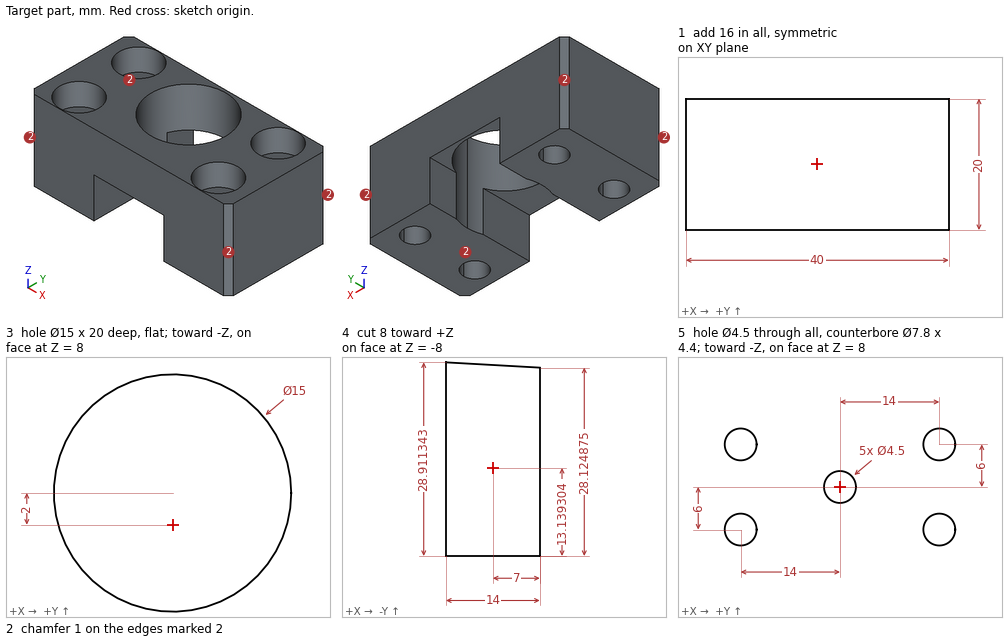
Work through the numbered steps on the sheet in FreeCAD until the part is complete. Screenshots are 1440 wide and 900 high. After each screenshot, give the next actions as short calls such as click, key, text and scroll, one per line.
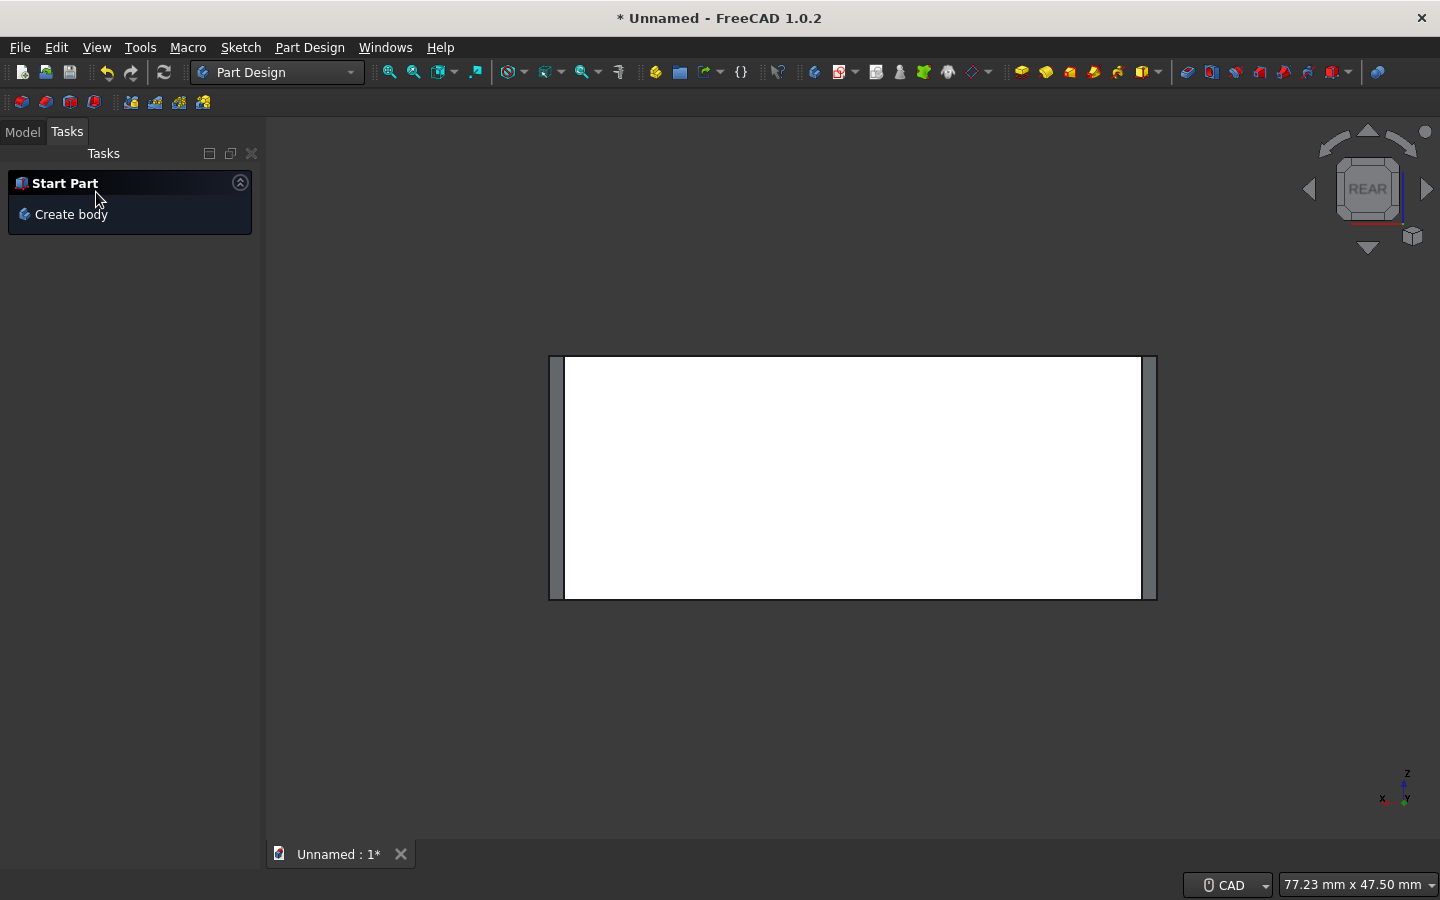
key(0)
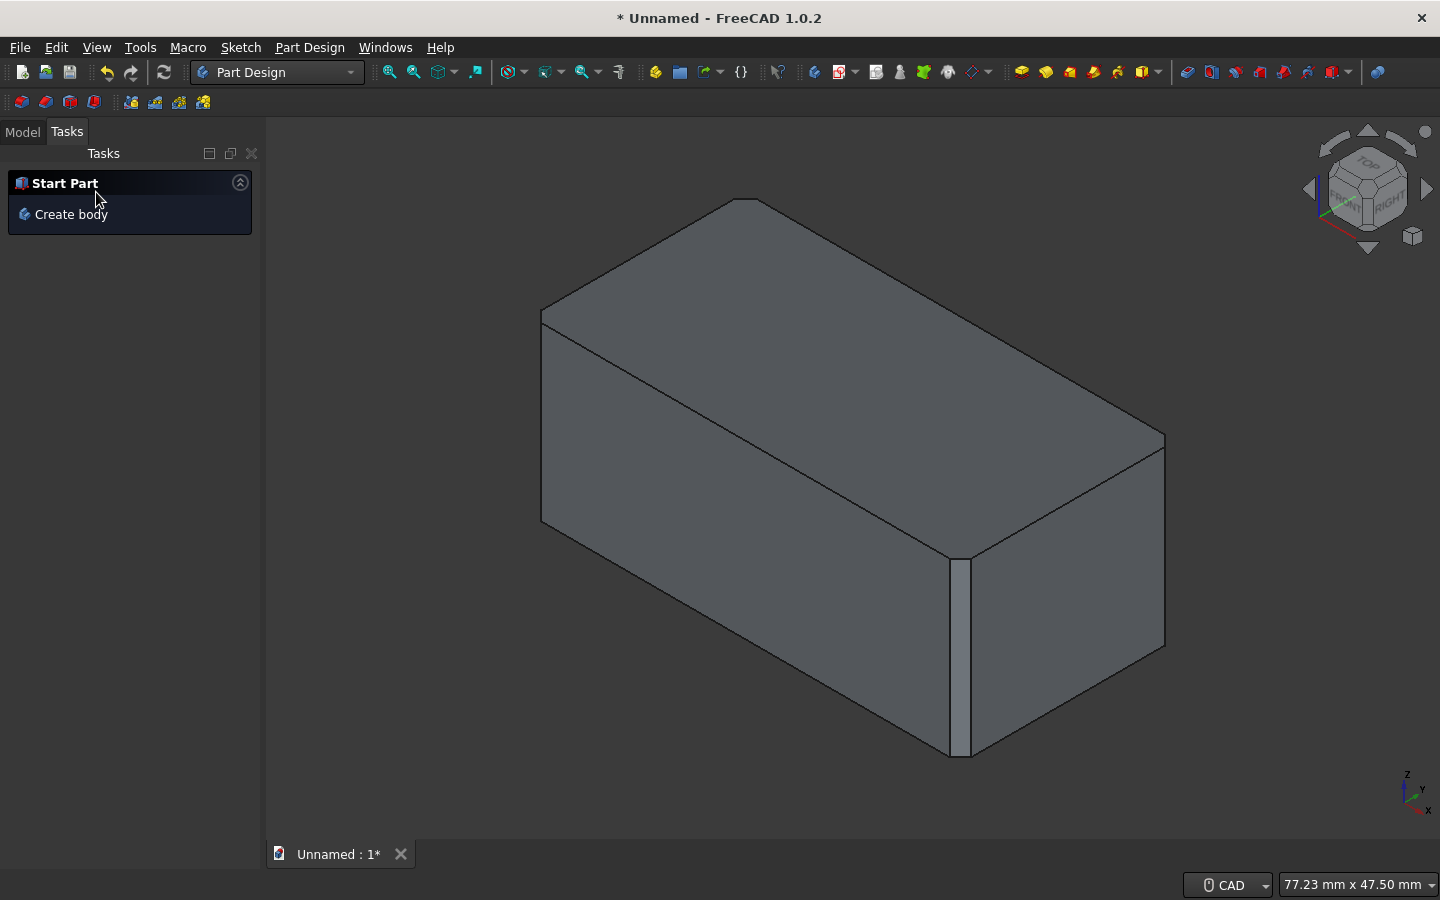
click(914, 413)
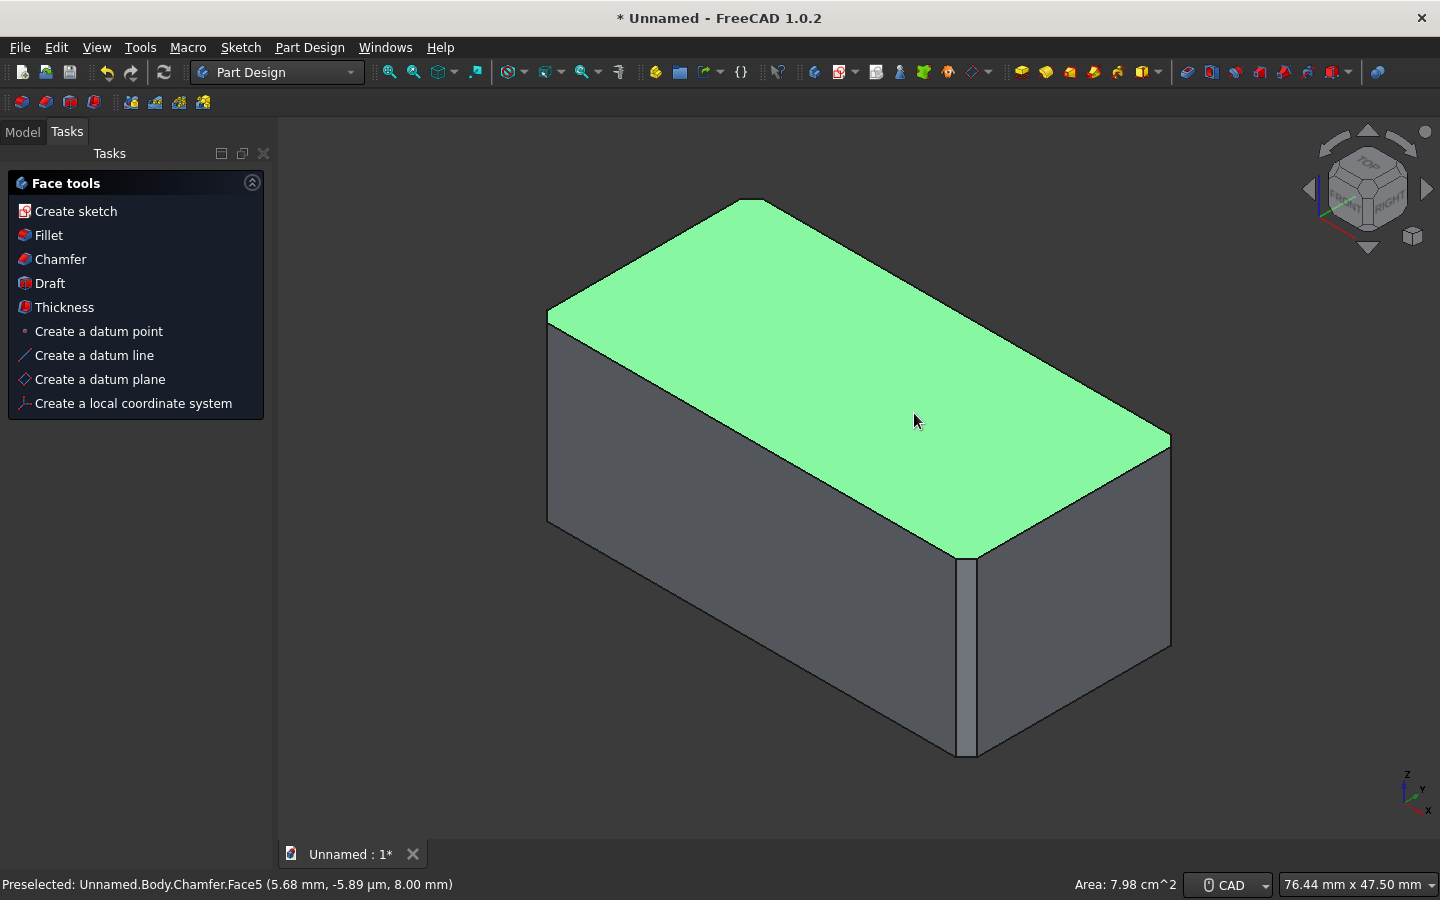
click(840, 72)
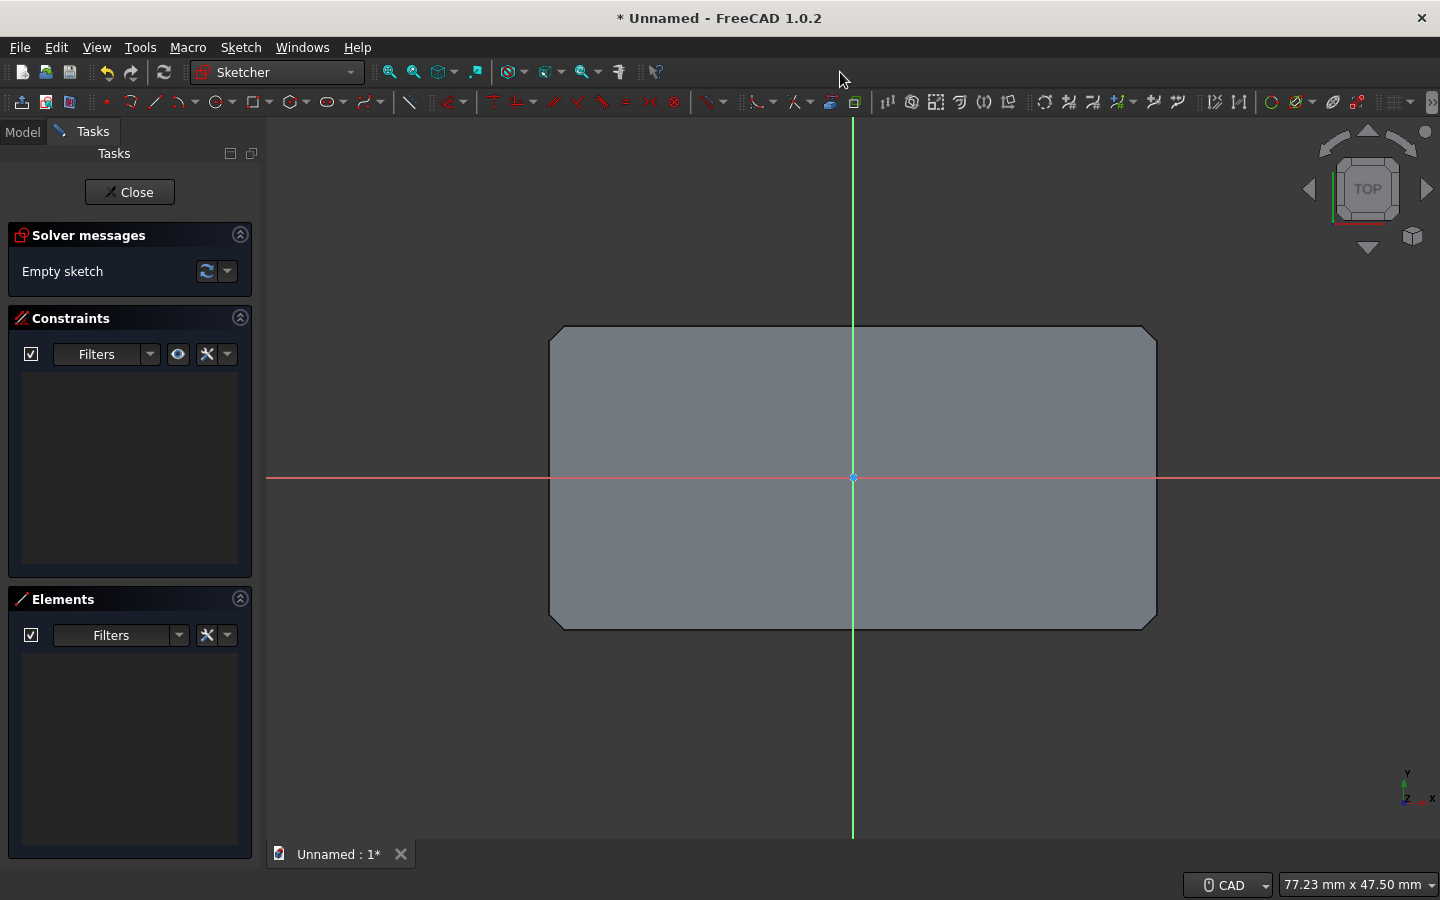
scroll(909, 423, up, 4)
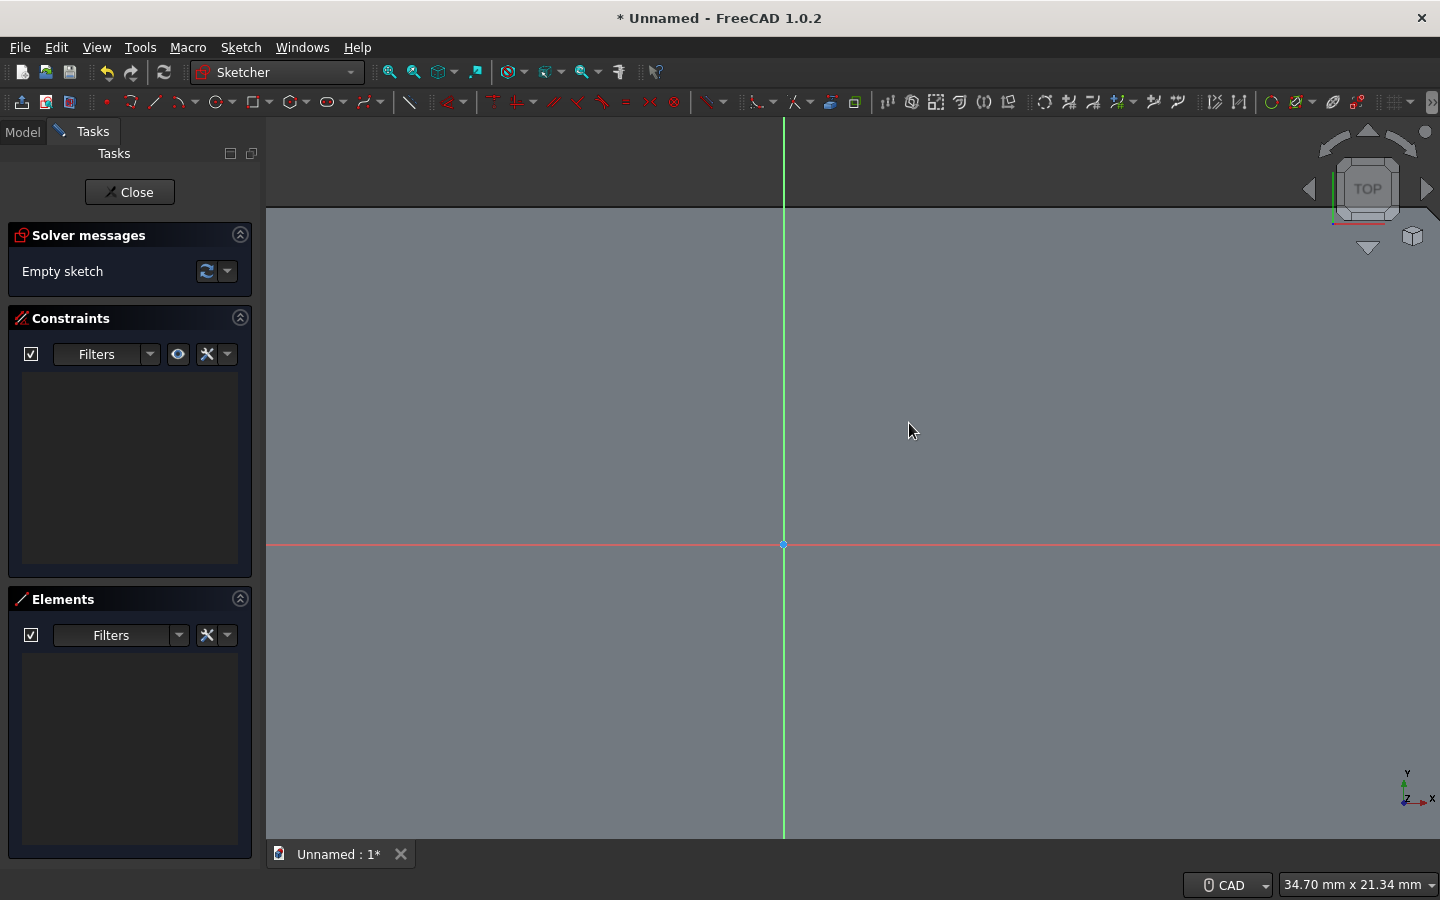
click(216, 102)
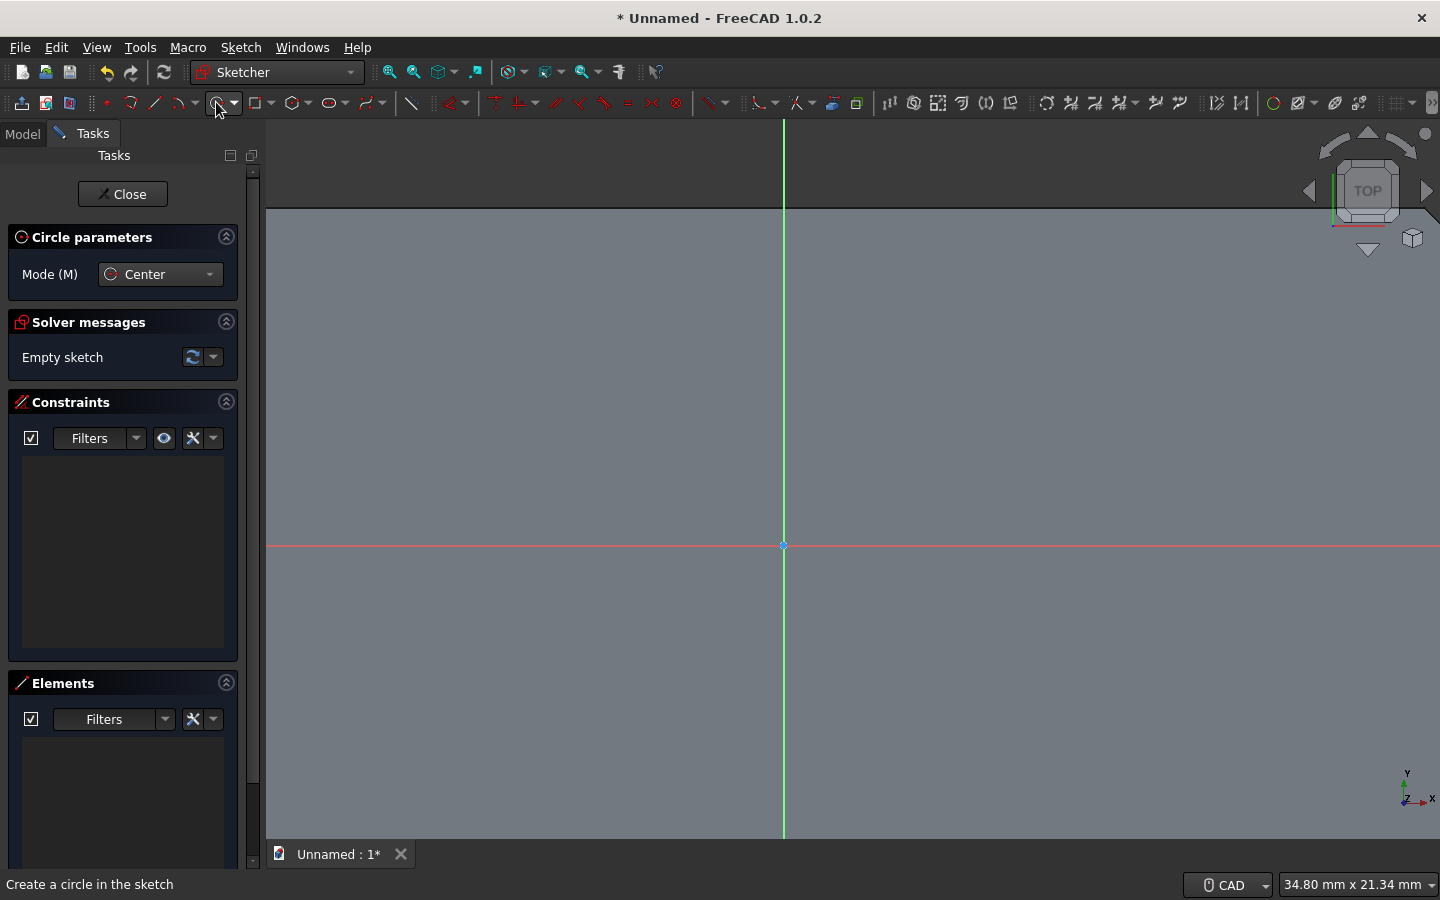
click(784, 478)
click(963, 299)
key(Escape)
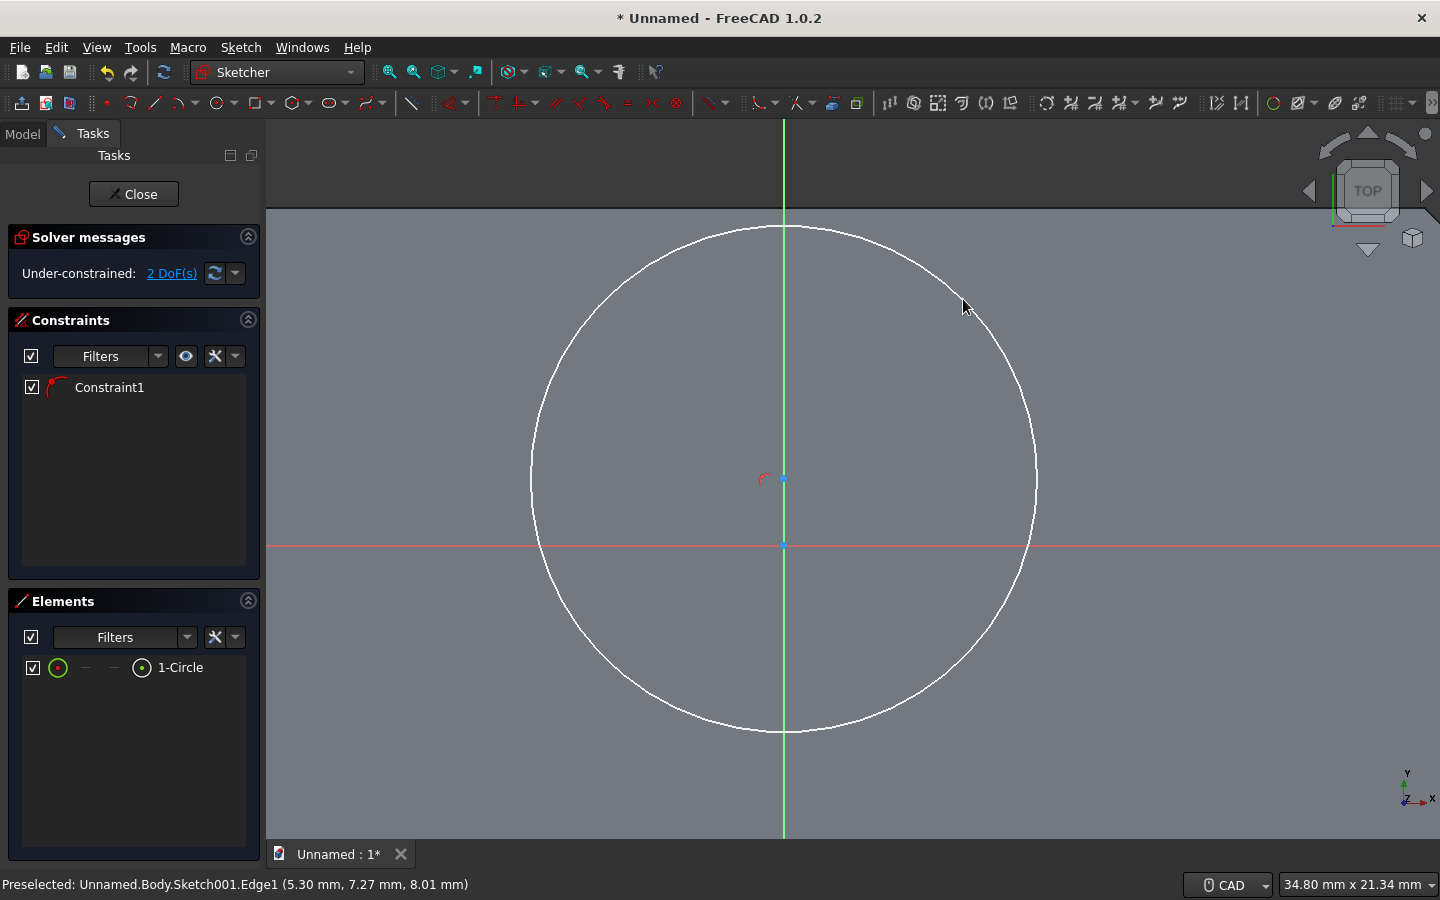
key(d)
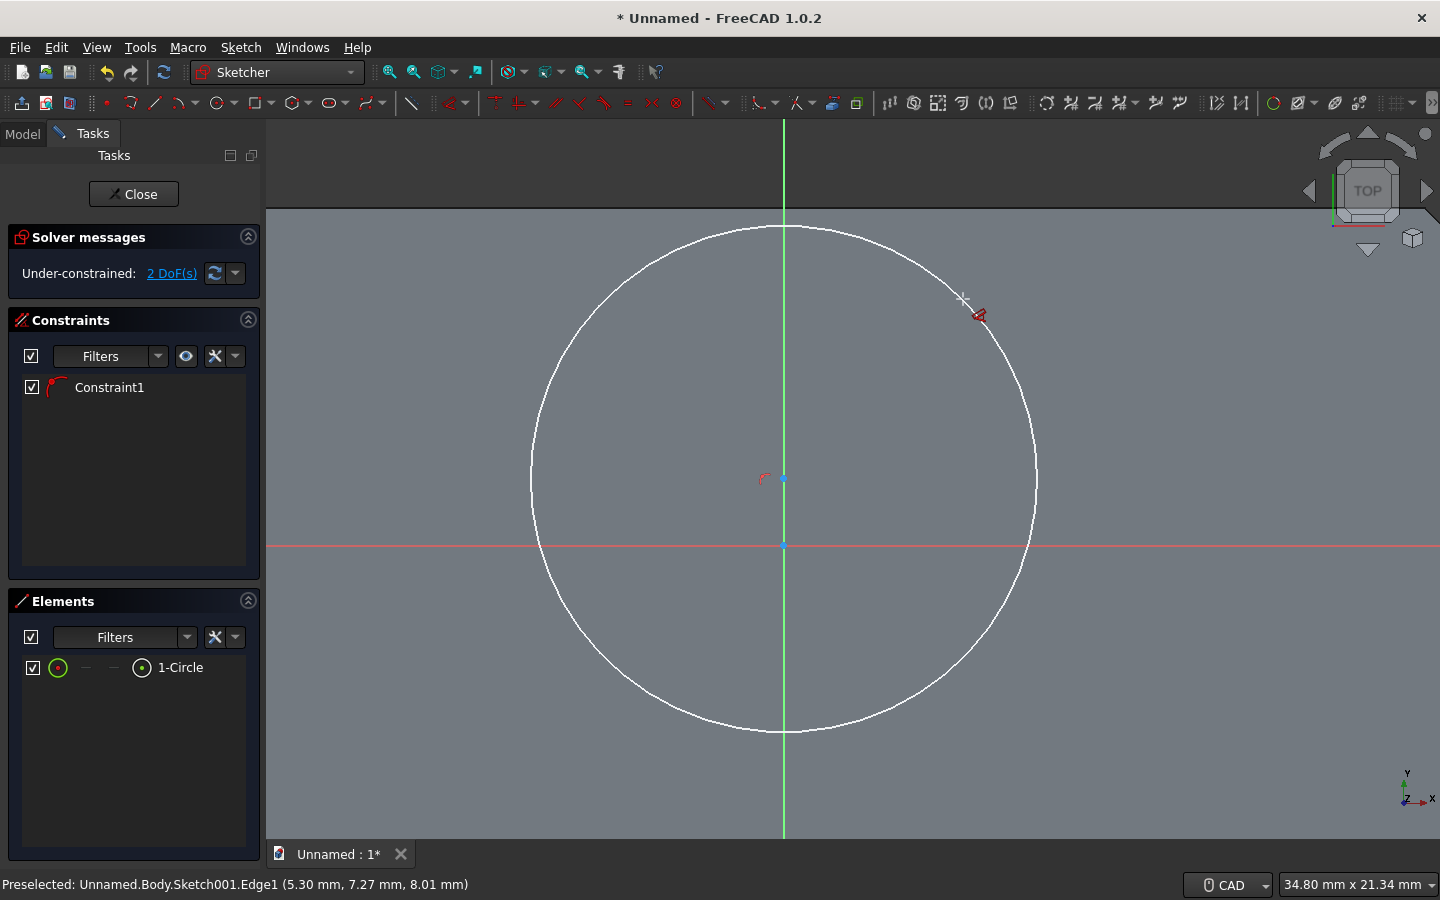
click(962, 299)
click(985, 276)